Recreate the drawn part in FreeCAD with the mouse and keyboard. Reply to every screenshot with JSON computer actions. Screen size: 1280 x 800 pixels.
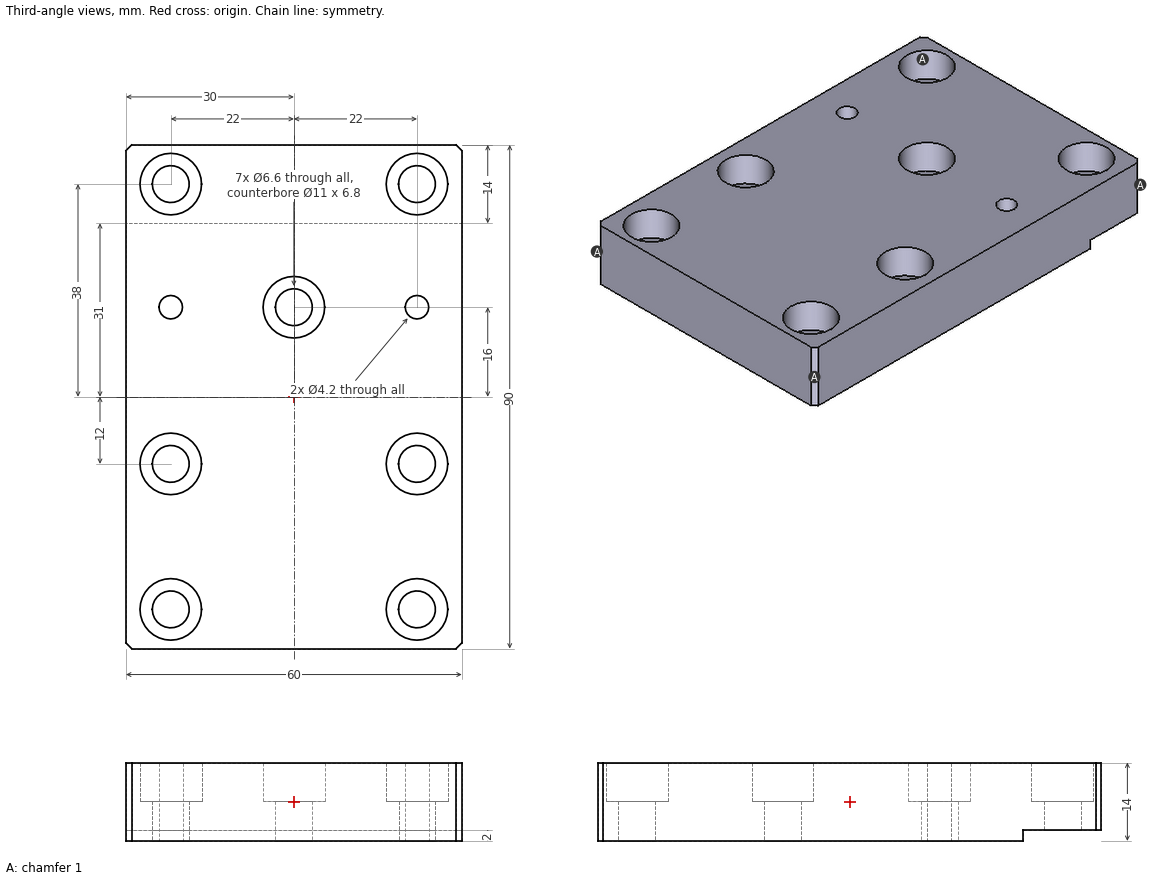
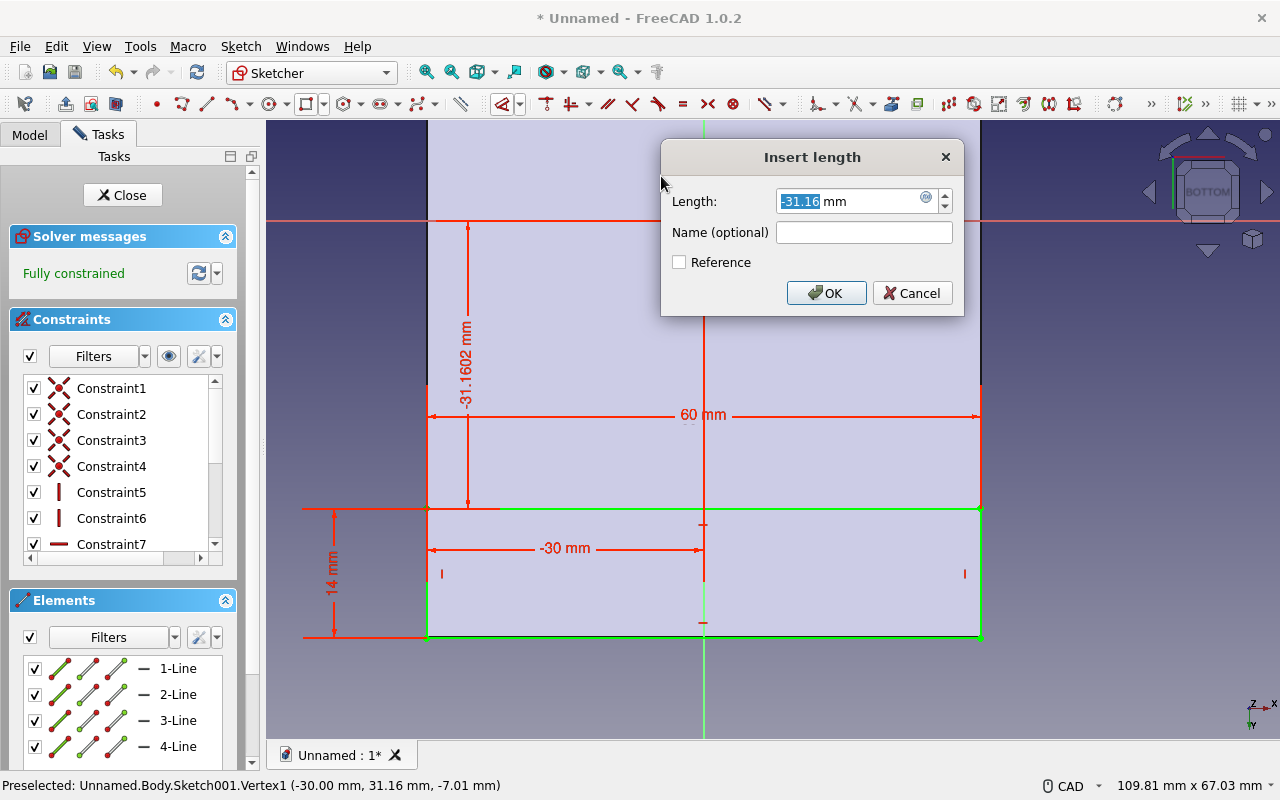
{"action": "type", "text": "-31"}
{"action": "key", "text": "Return"}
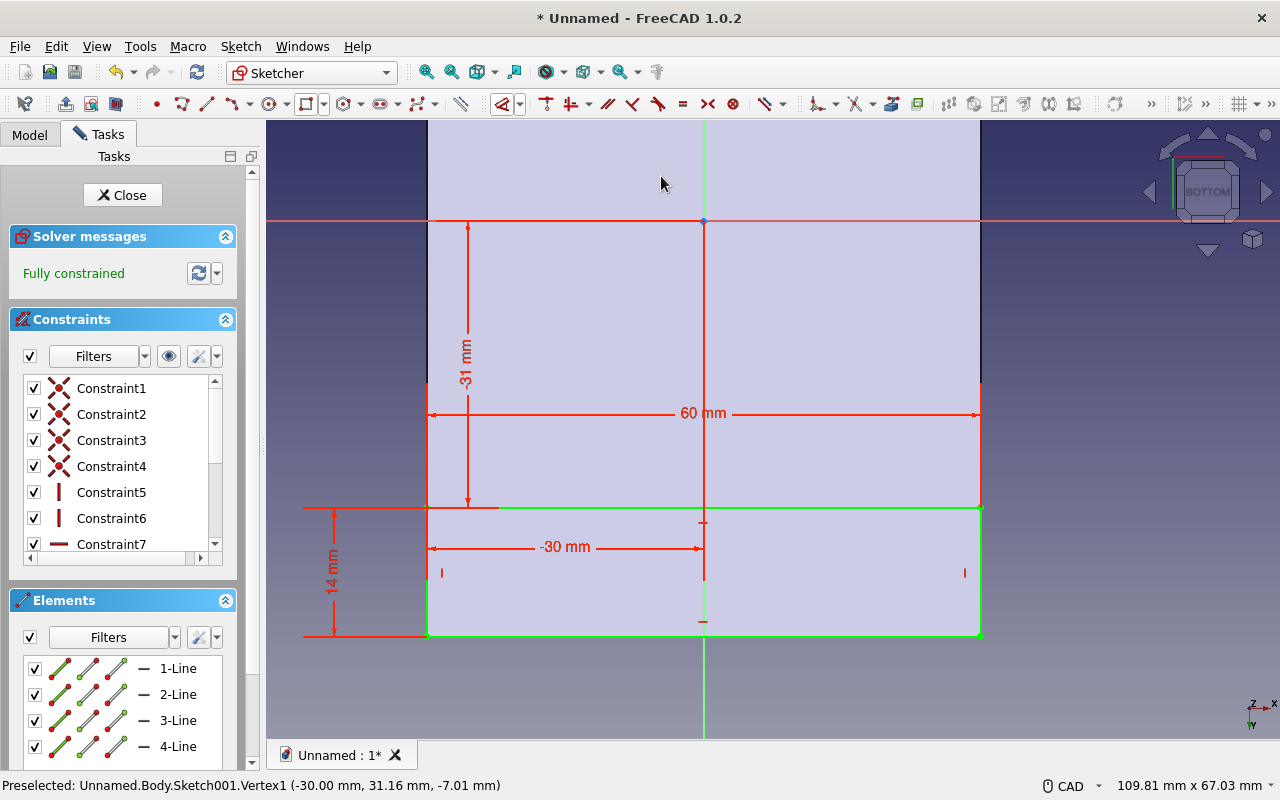
{"action": "left_click", "coordinate": [123, 195]}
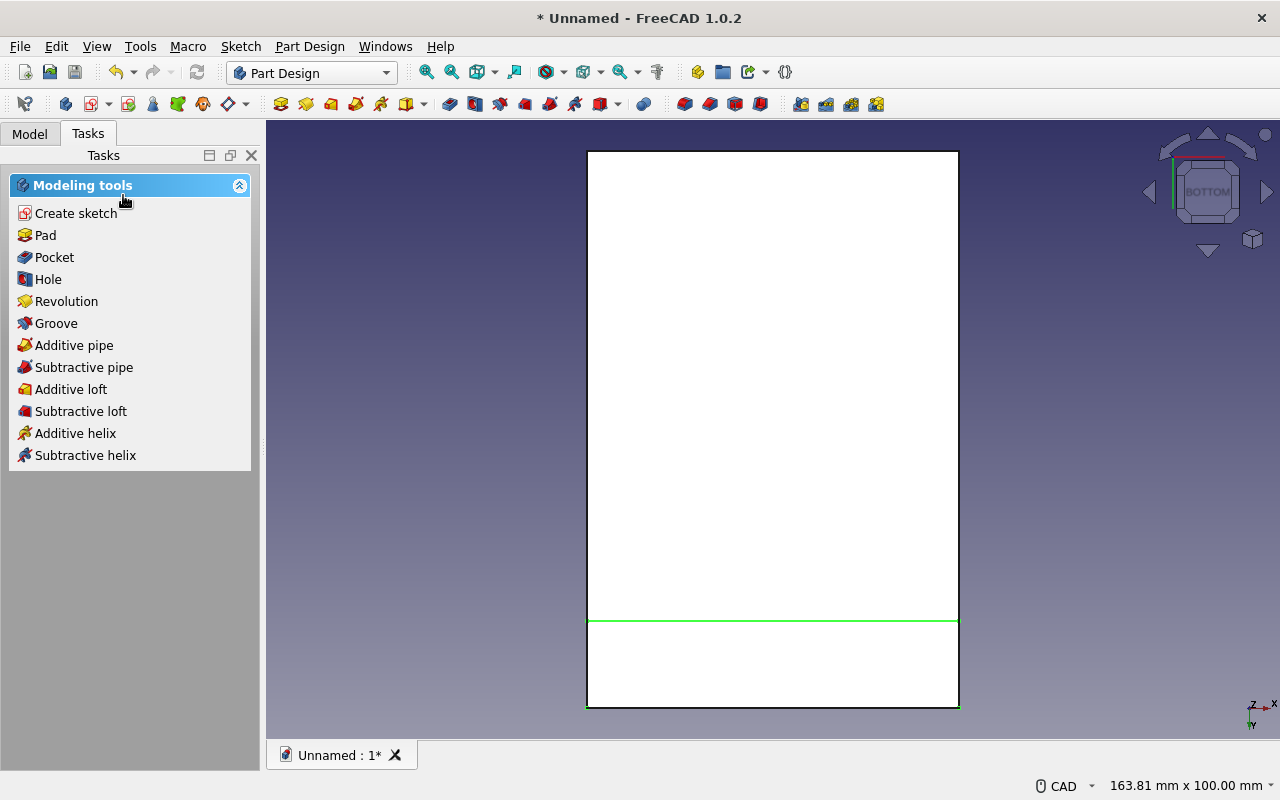
{"action": "left_click", "coordinate": [450, 104]}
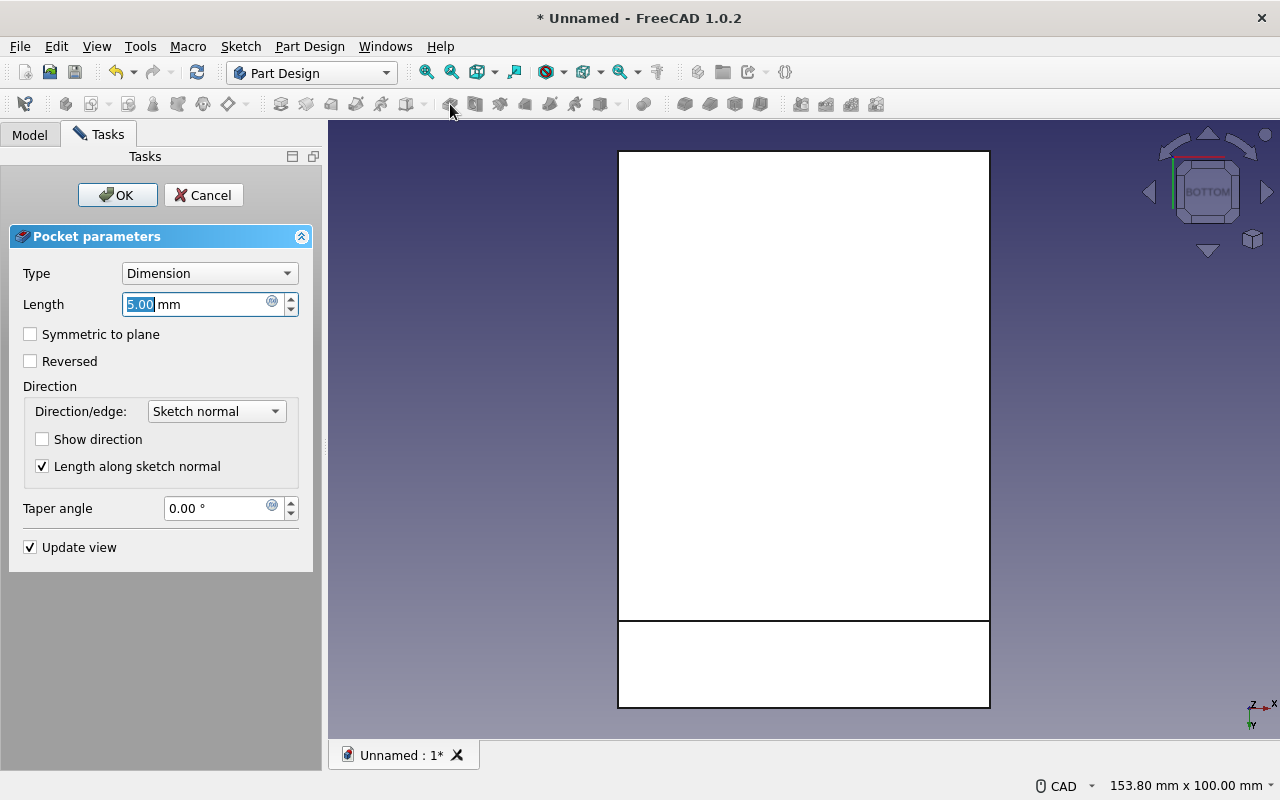
{"action": "type", "text": "2"}
{"action": "key", "text": "Tab"}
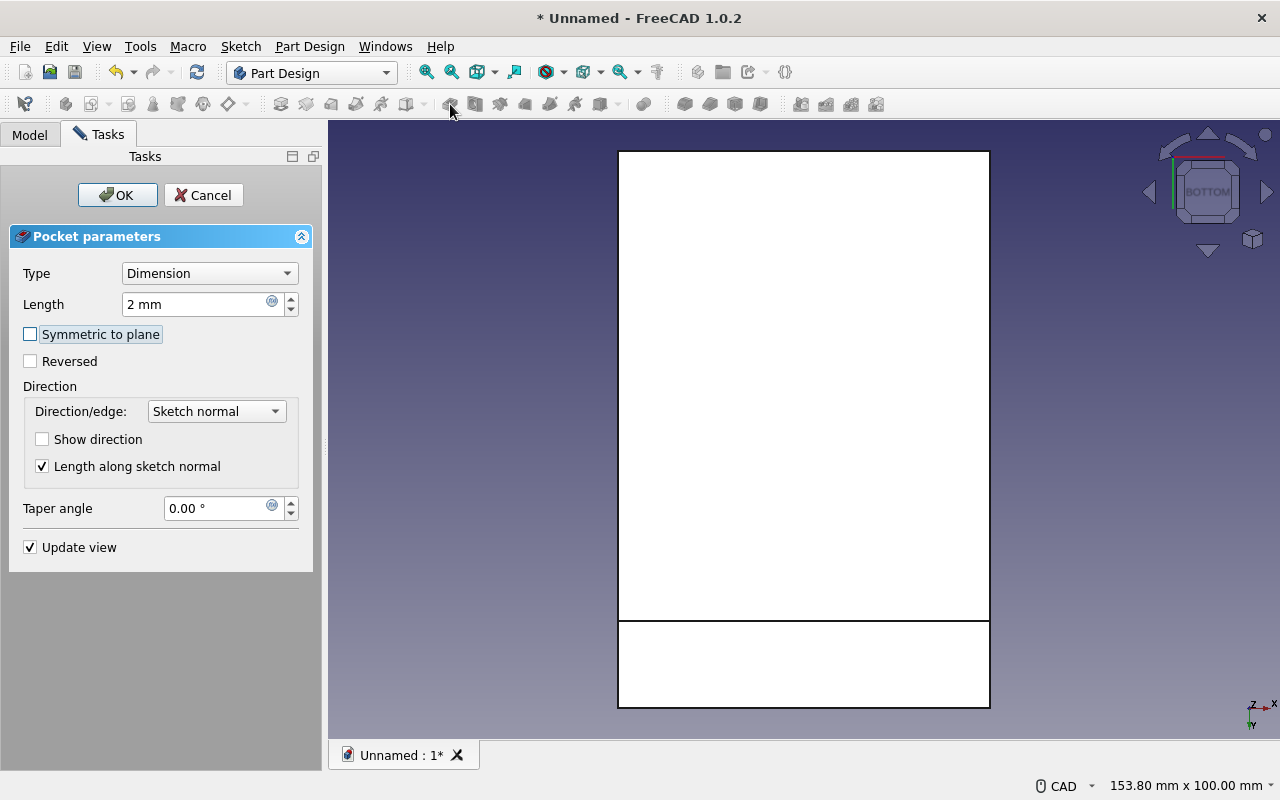
{"action": "left_click", "coordinate": [118, 195]}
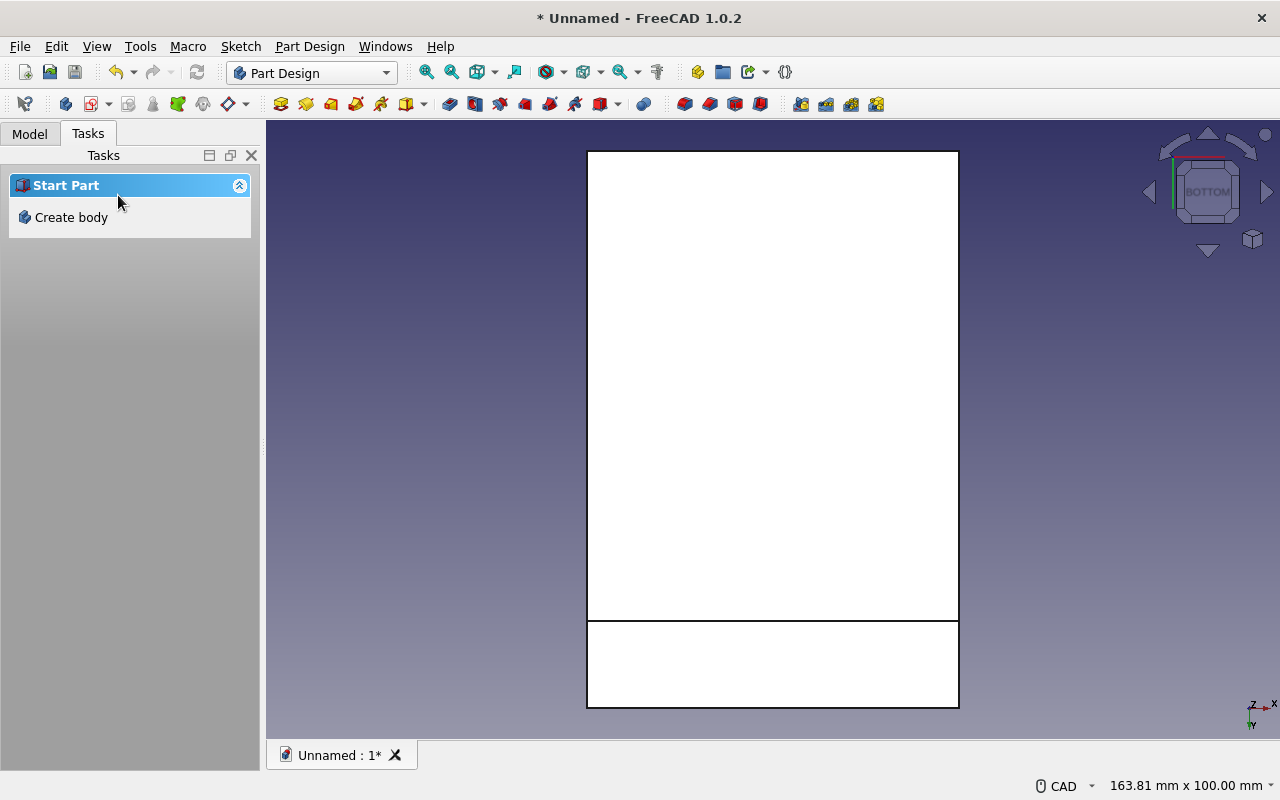
{"action": "key", "text": "0"}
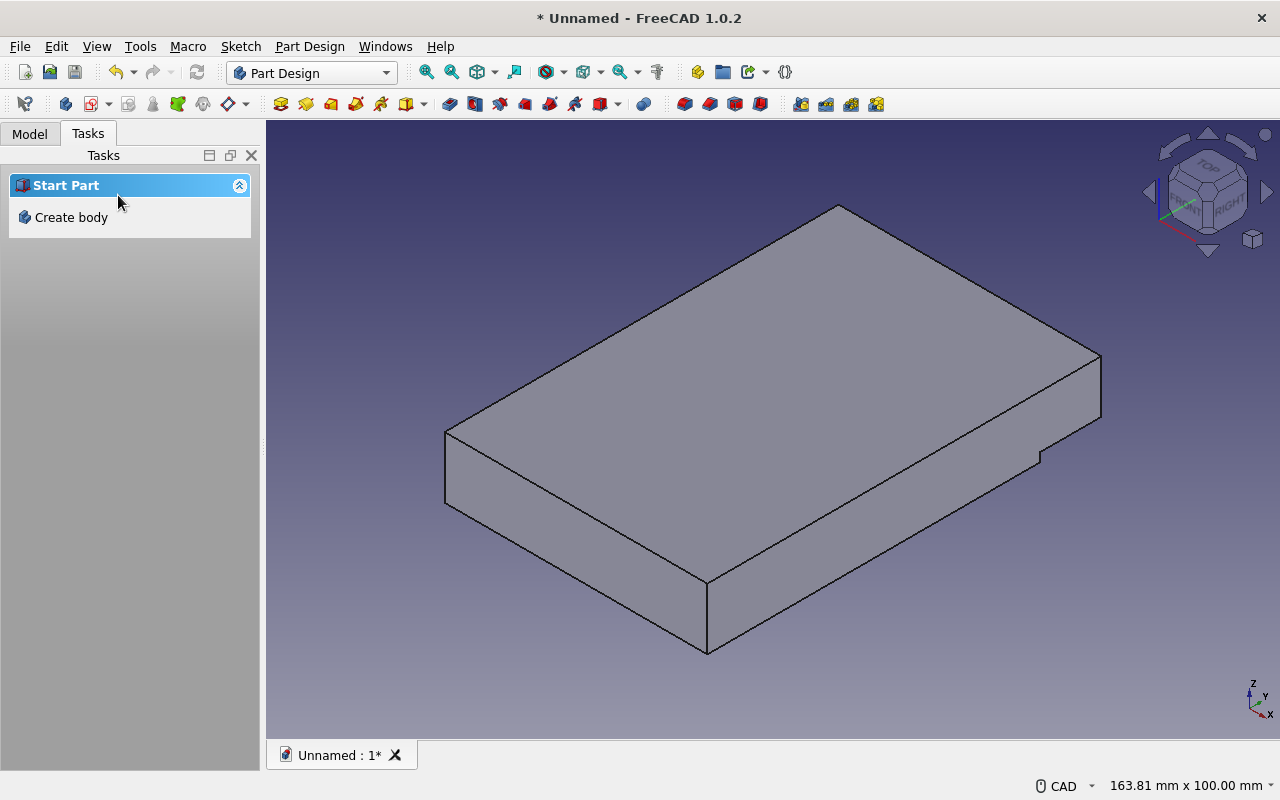
{"action": "left_click", "coordinate": [829, 361]}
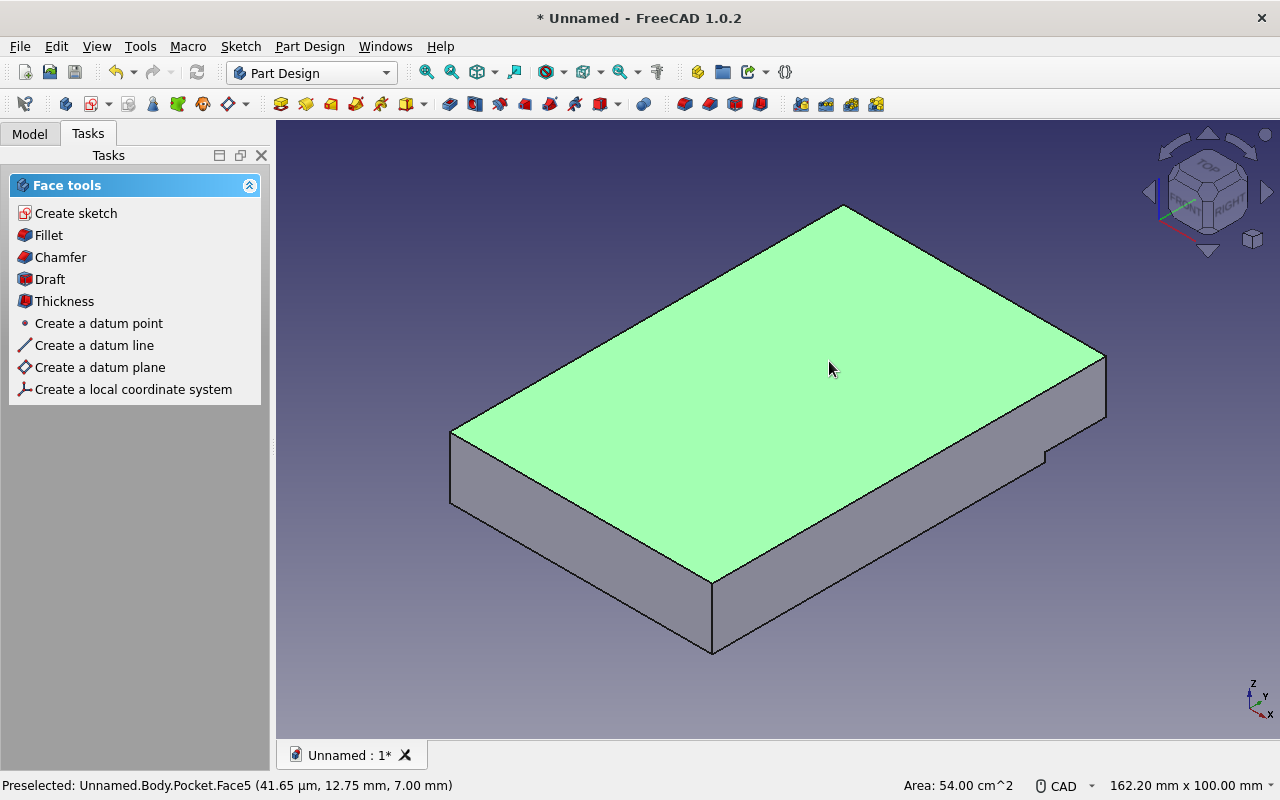
{"action": "left_click", "coordinate": [90, 104]}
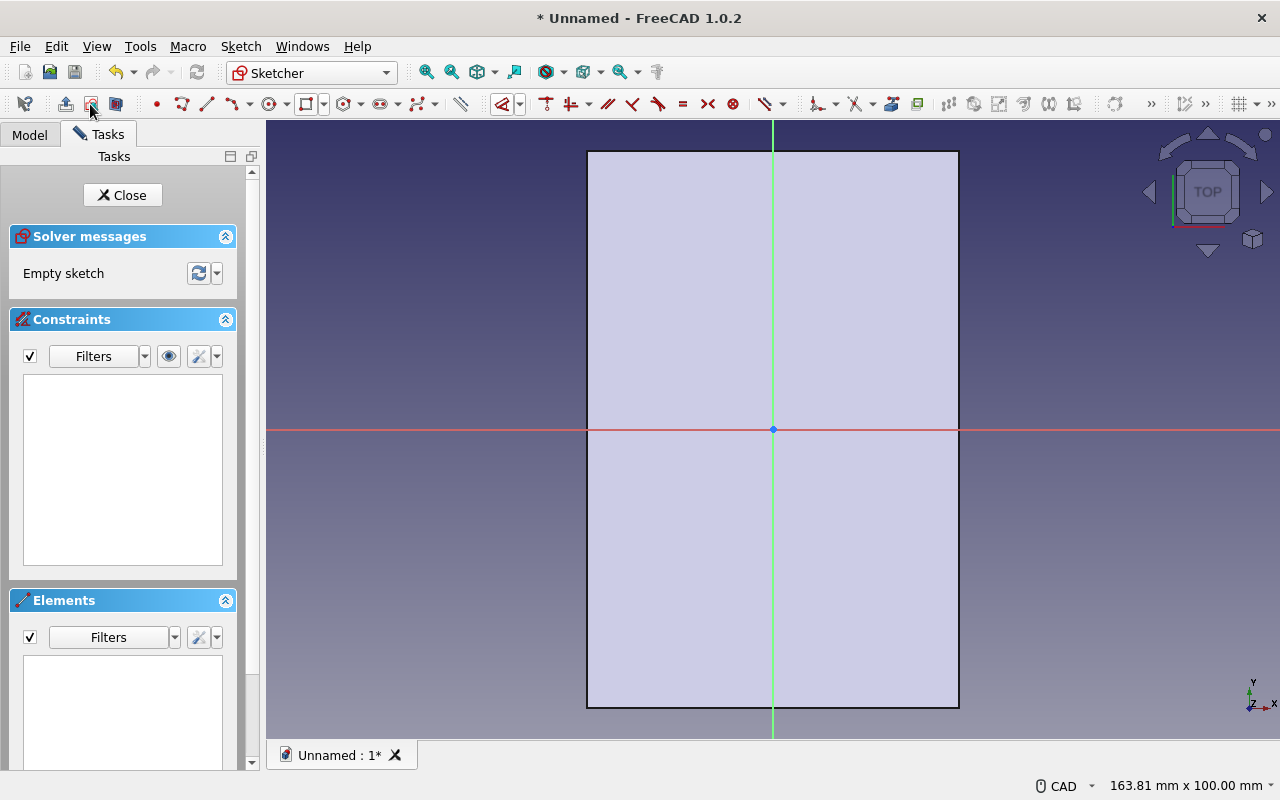
{"action": "left_click", "coordinate": [268, 104]}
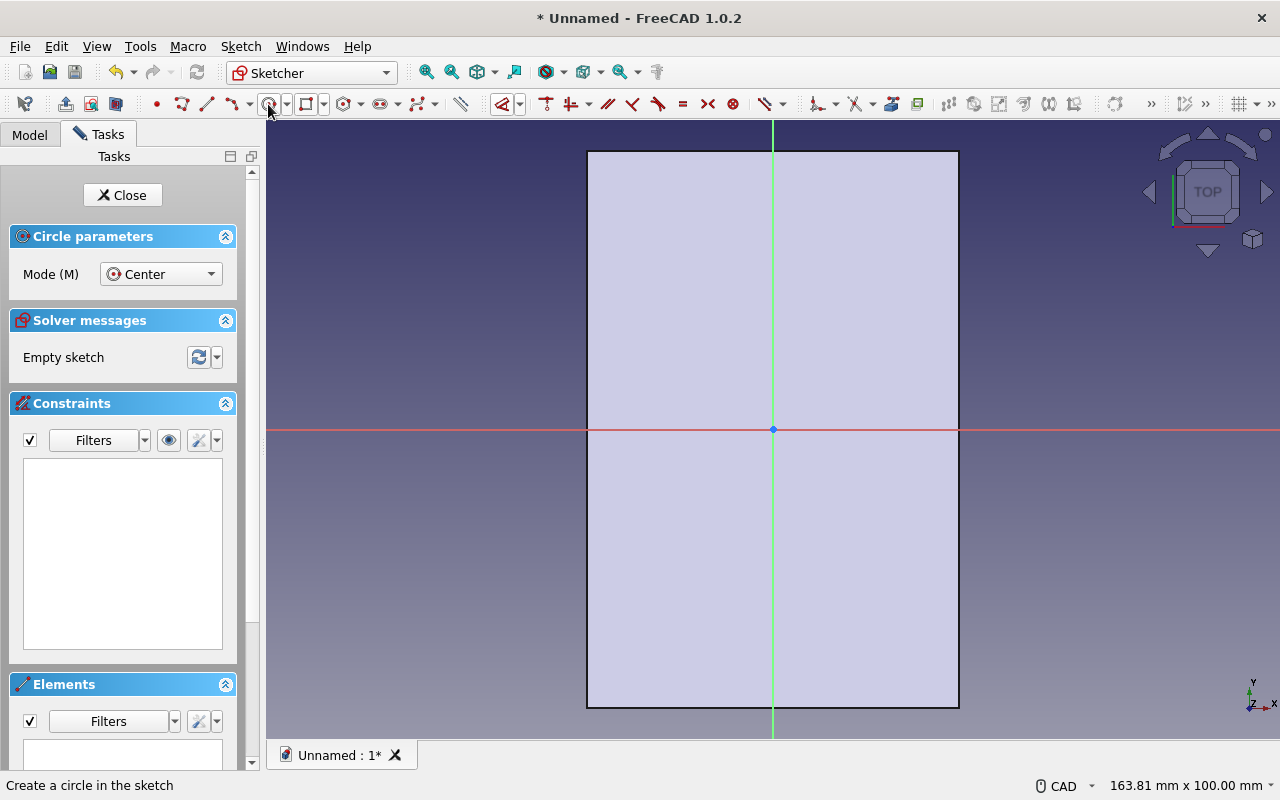
{"action": "left_click", "coordinate": [773, 330]}
{"action": "mouse_move", "coordinate": [787, 316]}